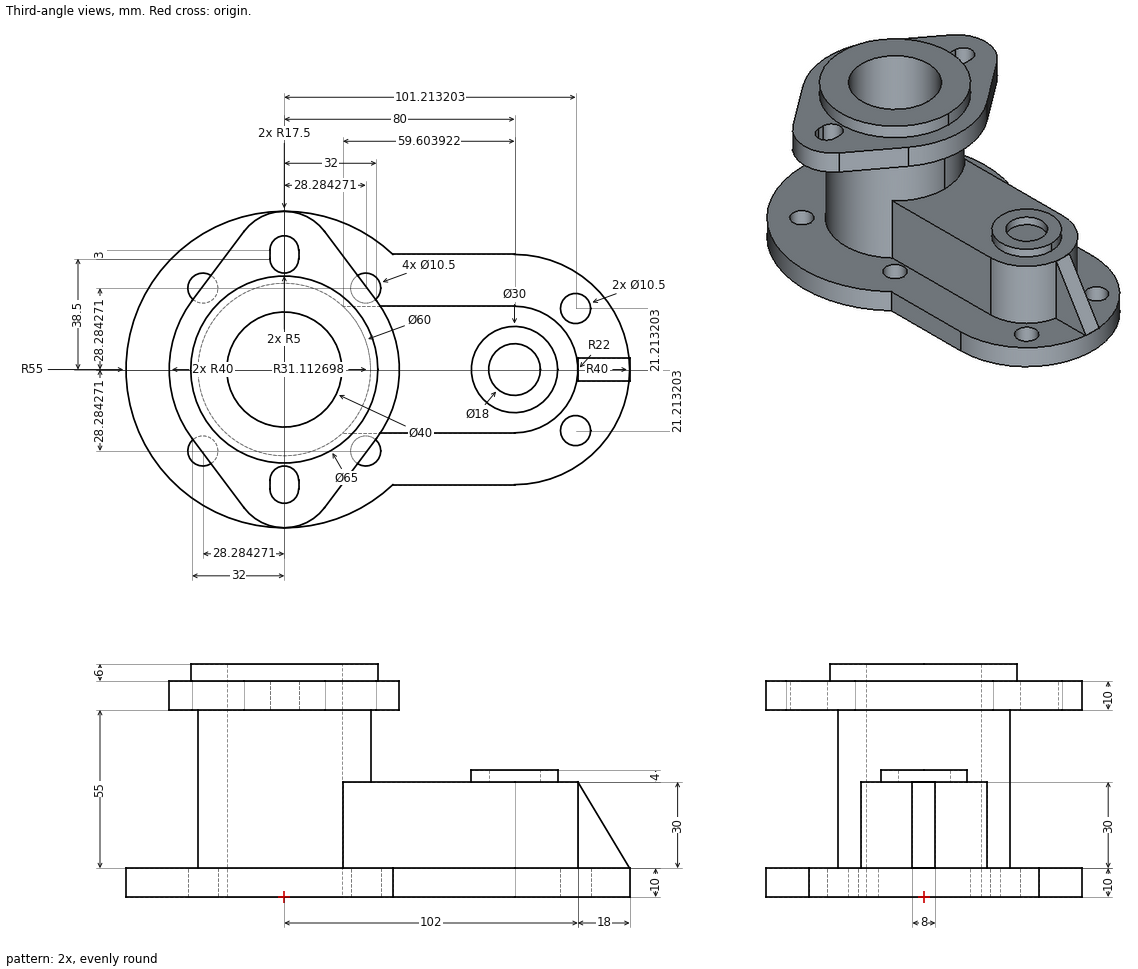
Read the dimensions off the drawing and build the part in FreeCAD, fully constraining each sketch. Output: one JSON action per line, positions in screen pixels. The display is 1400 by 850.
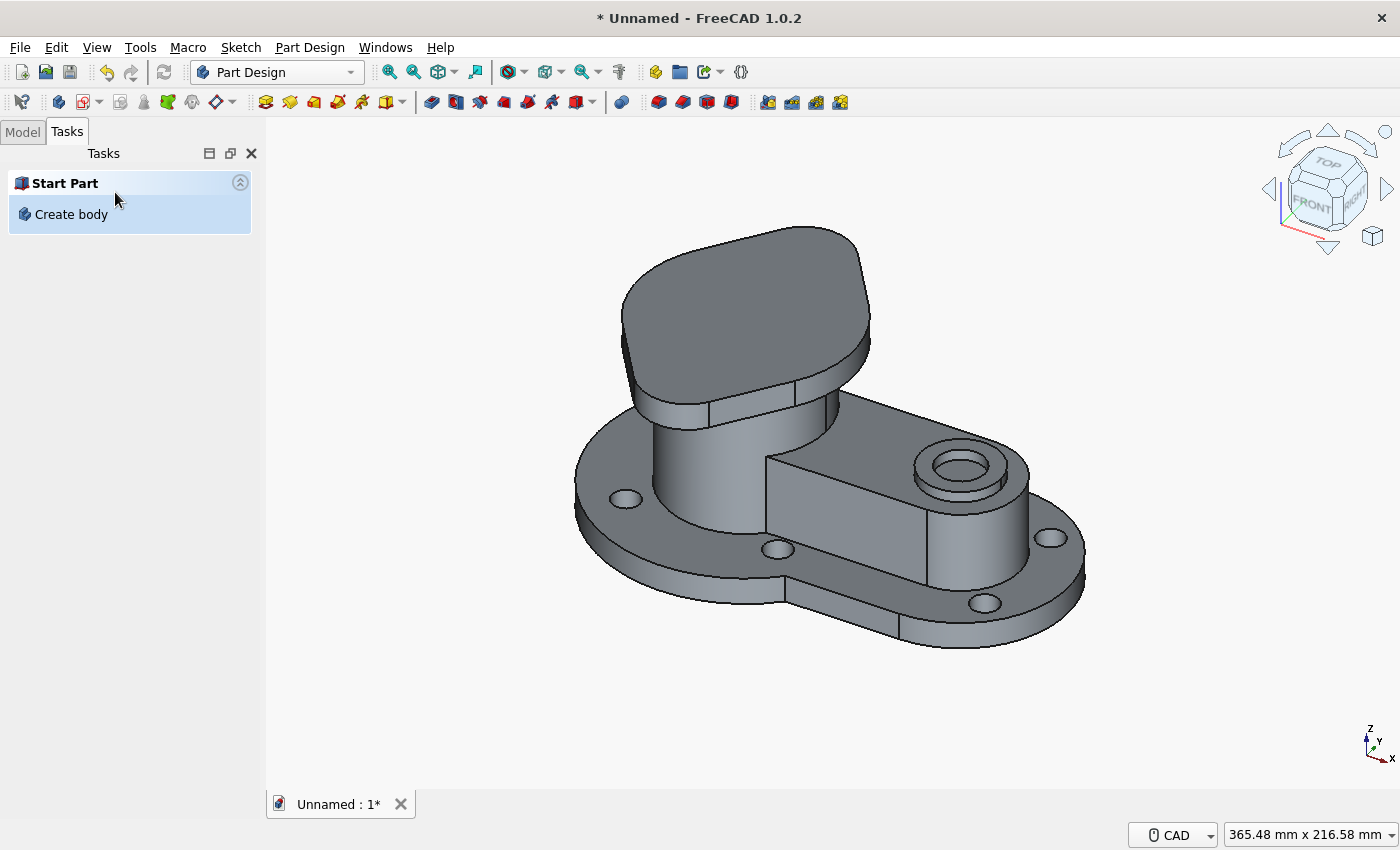
{"action": "left_click", "coordinate": [746, 315]}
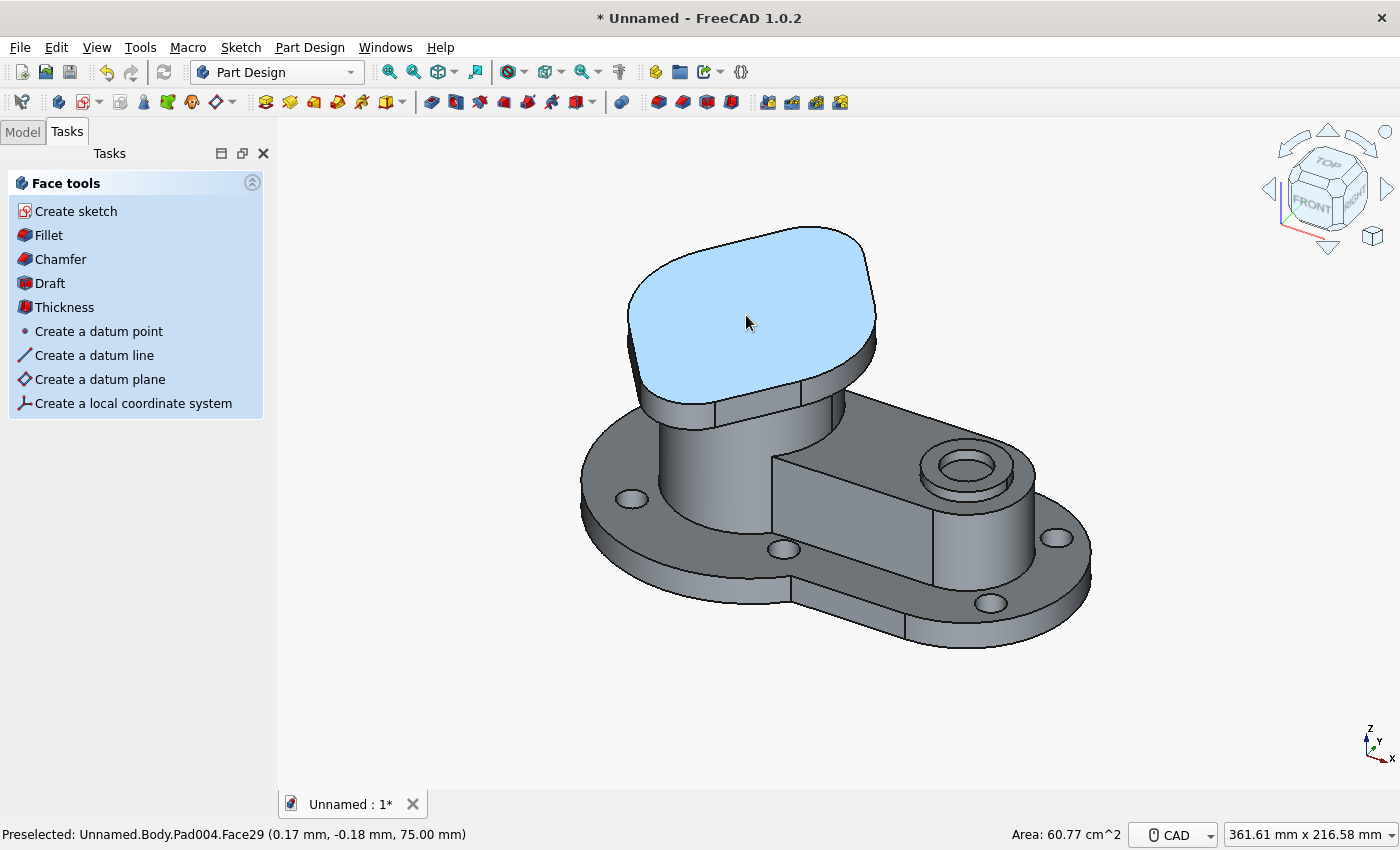
{"action": "left_click", "coordinate": [84, 102]}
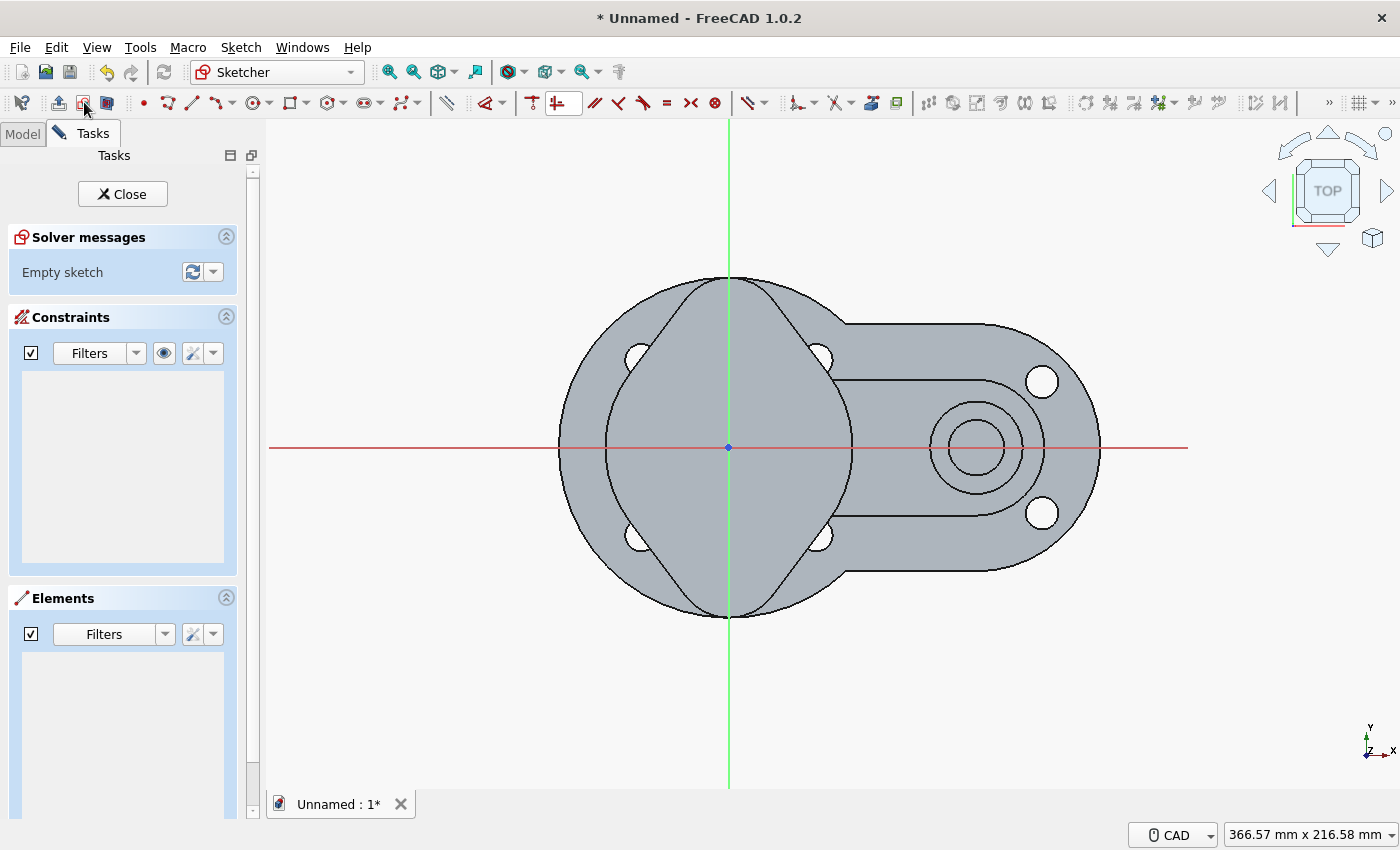
{"action": "scroll", "coordinate": [700, 442], "scroll_direction": "up", "scroll_amount": 4}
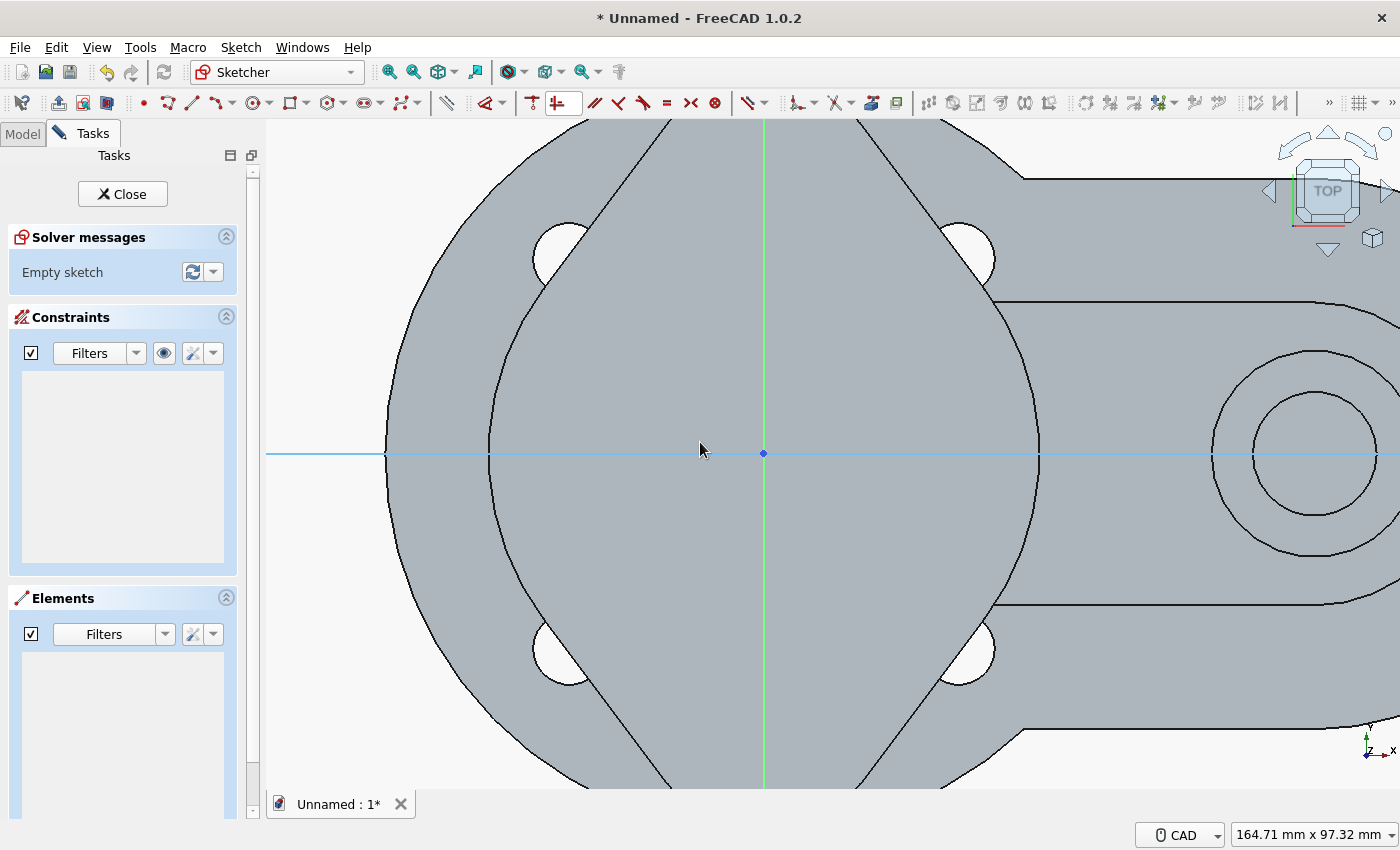
{"action": "key", "text": "g c"}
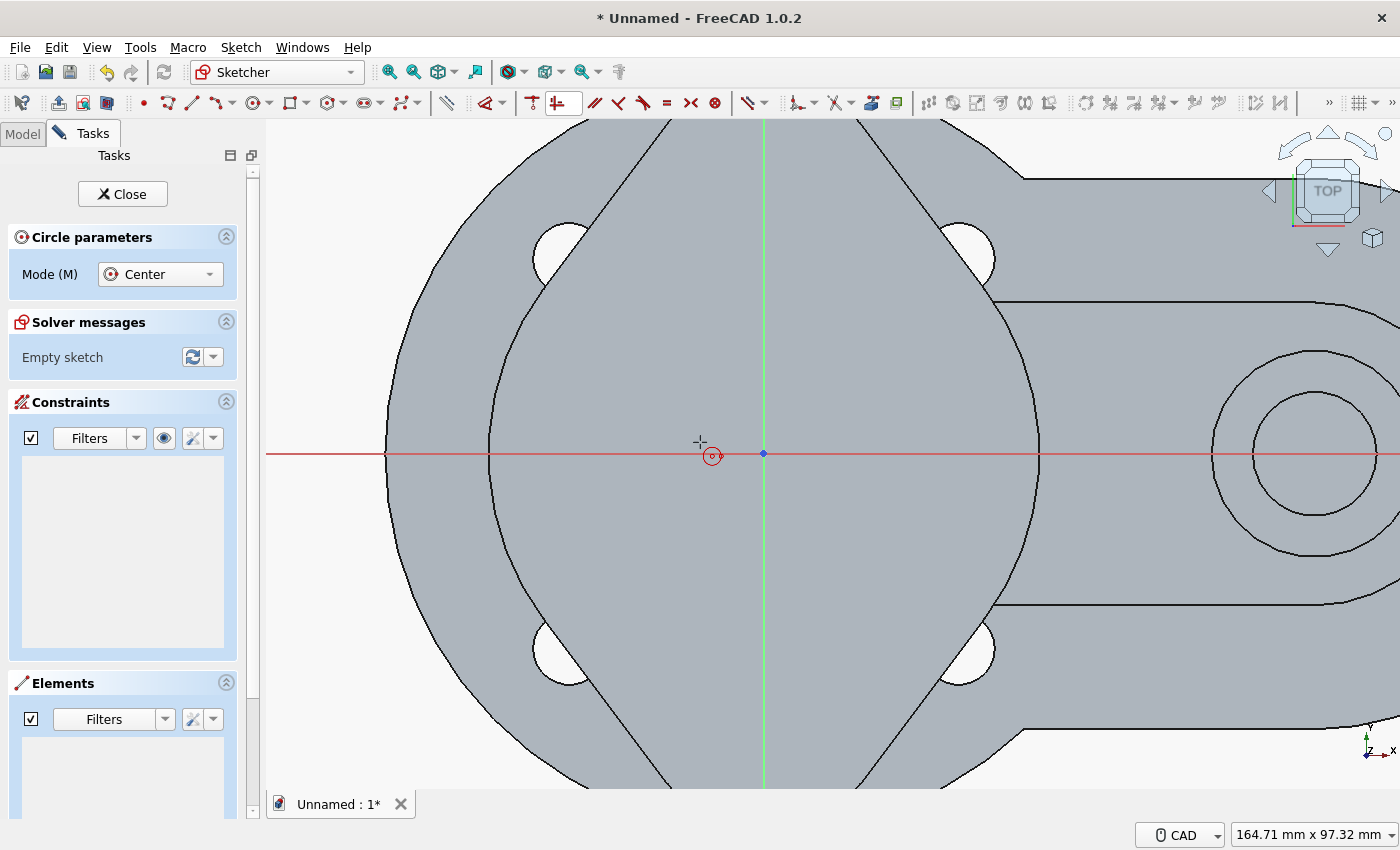
{"action": "left_click", "coordinate": [764, 454]}
{"action": "mouse_move", "coordinate": [922, 296]}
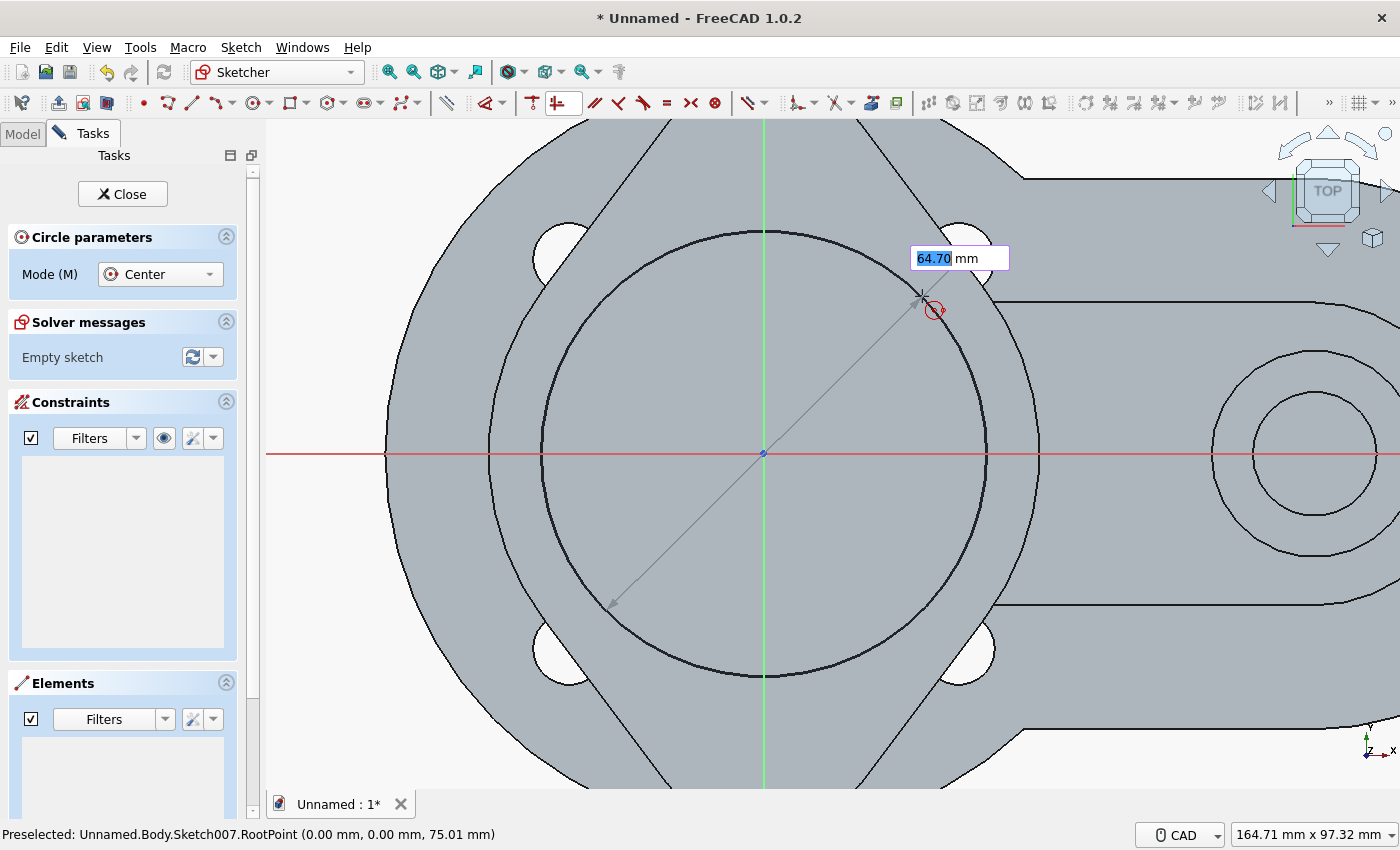
{"action": "type", "text": "65"}
{"action": "key", "text": "Return"}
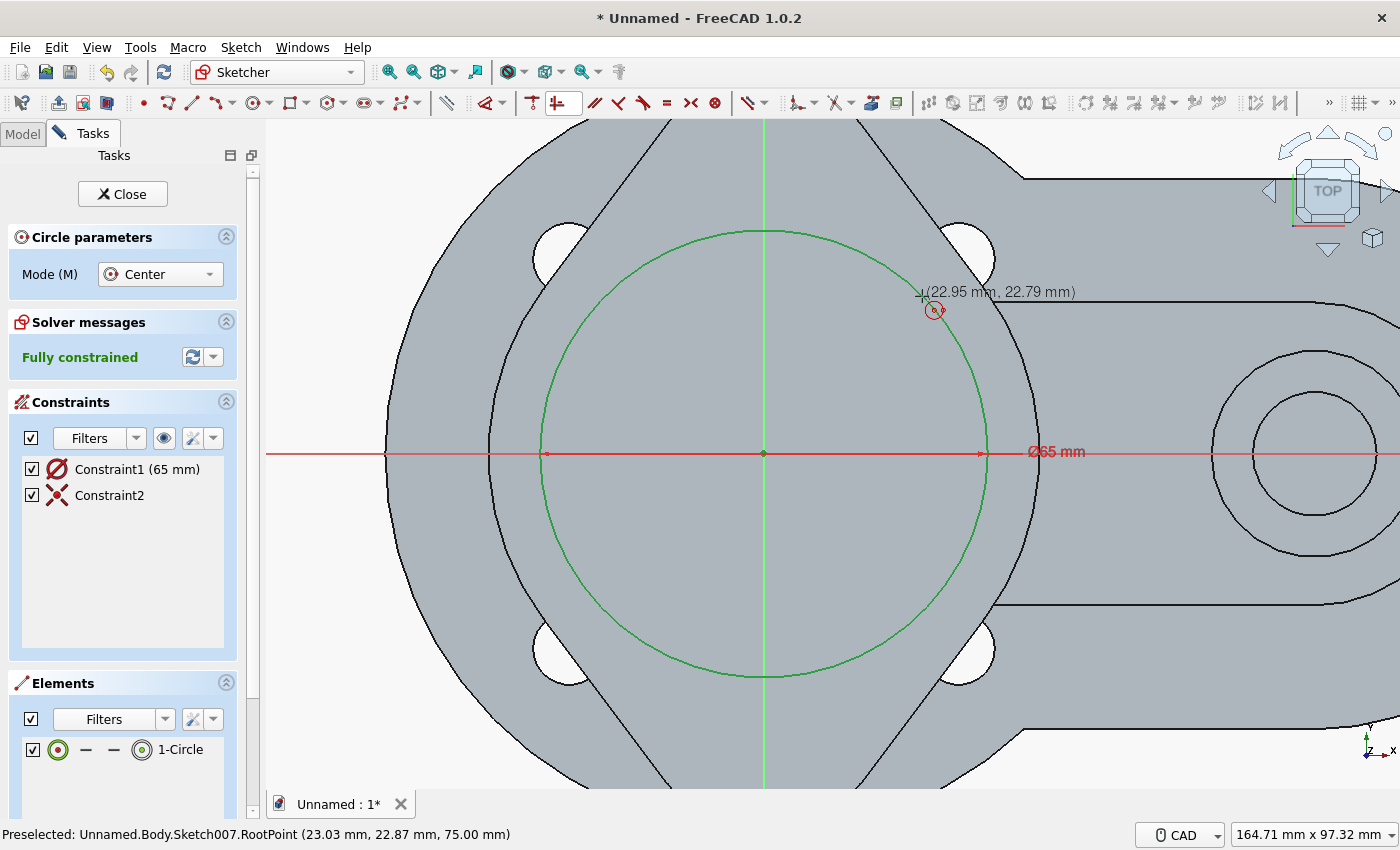
{"action": "left_click", "coordinate": [764, 454]}
{"action": "mouse_move", "coordinate": [861, 357]}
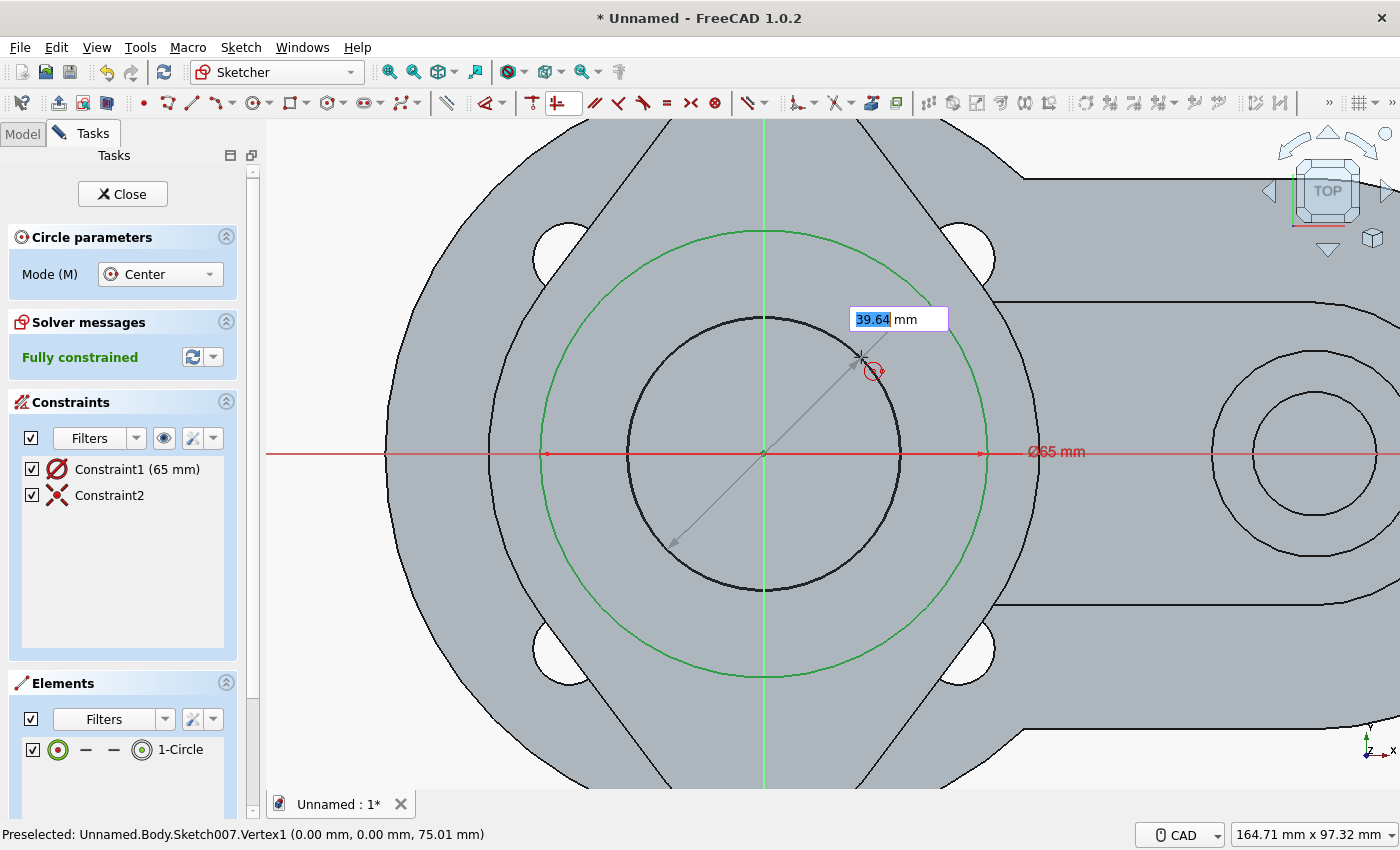
{"action": "type", "text": "40"}
{"action": "key", "text": "Return"}
{"action": "key", "text": "Escape"}